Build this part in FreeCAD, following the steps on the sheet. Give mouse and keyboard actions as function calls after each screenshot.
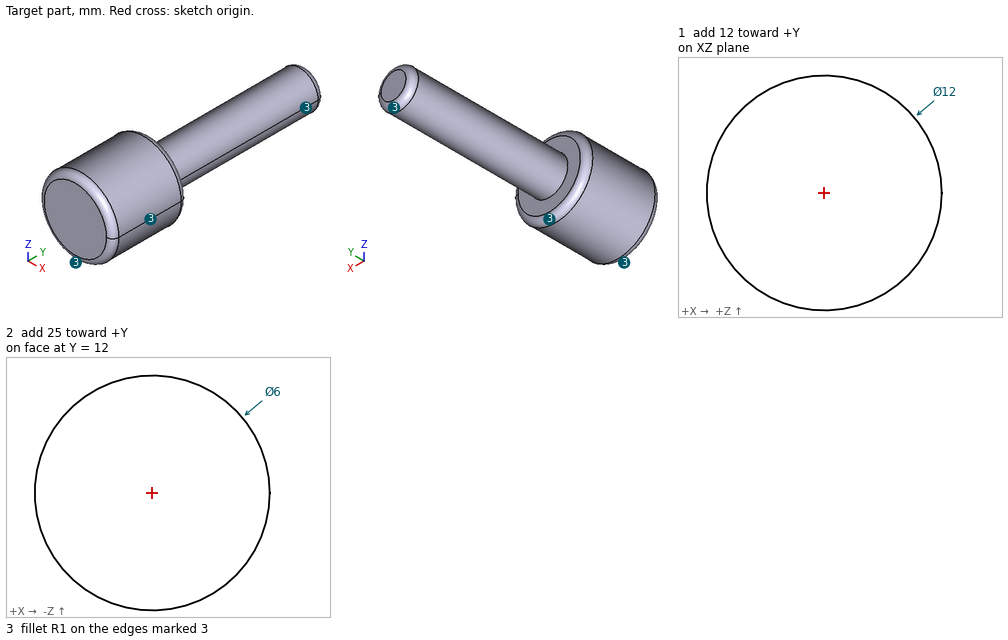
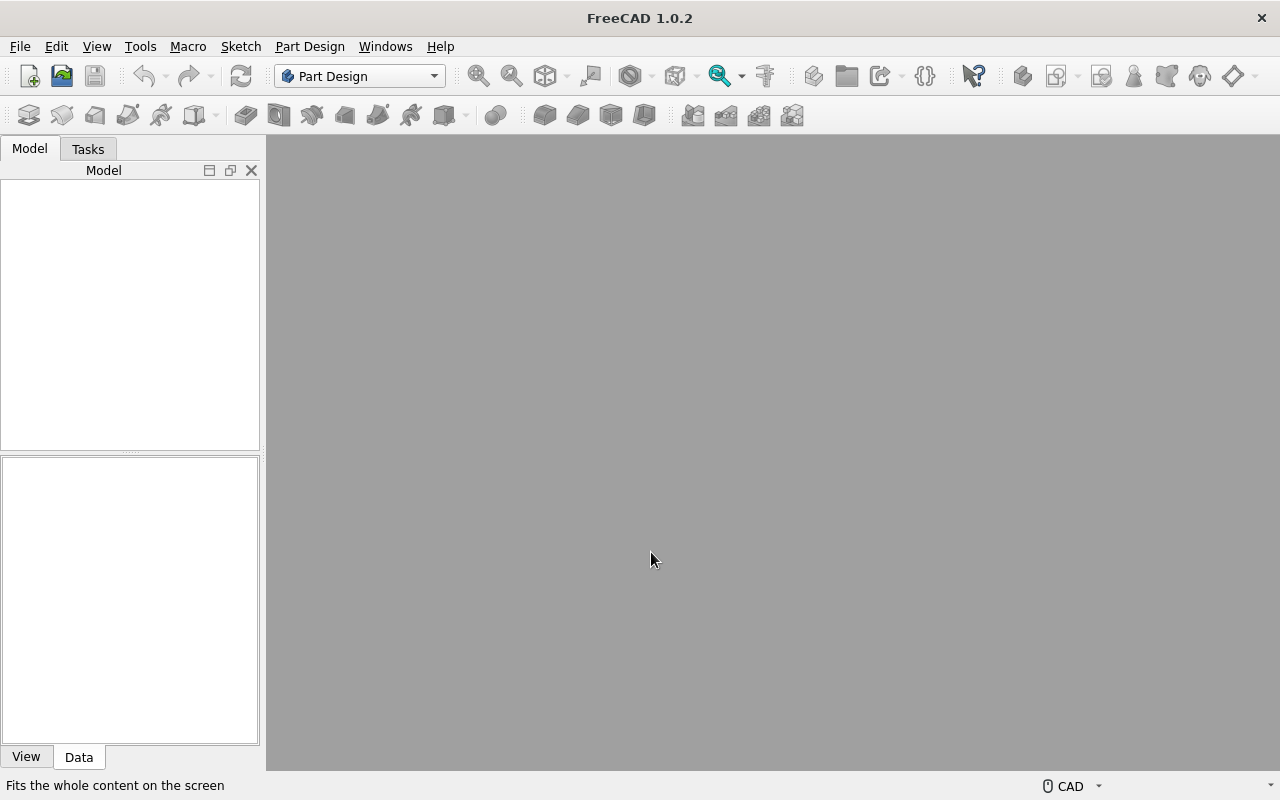
click(29, 76)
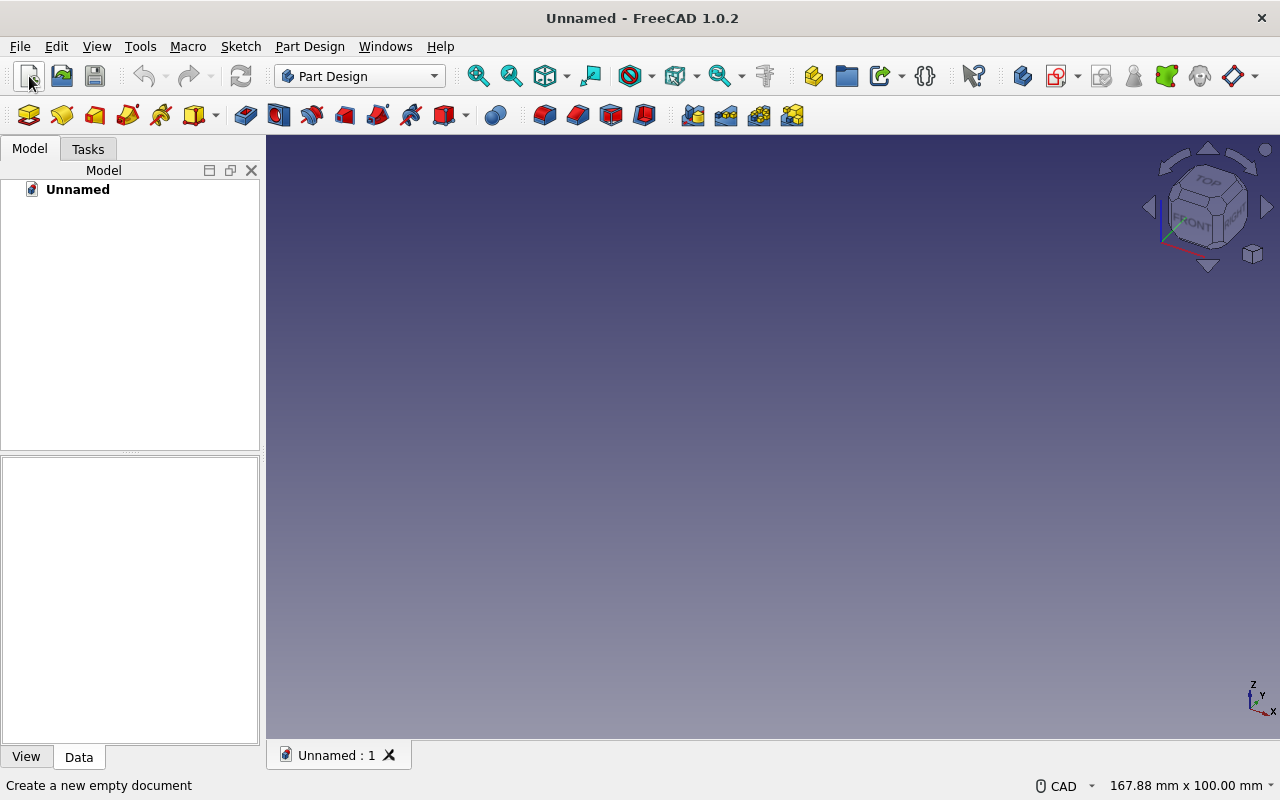
click(1056, 76)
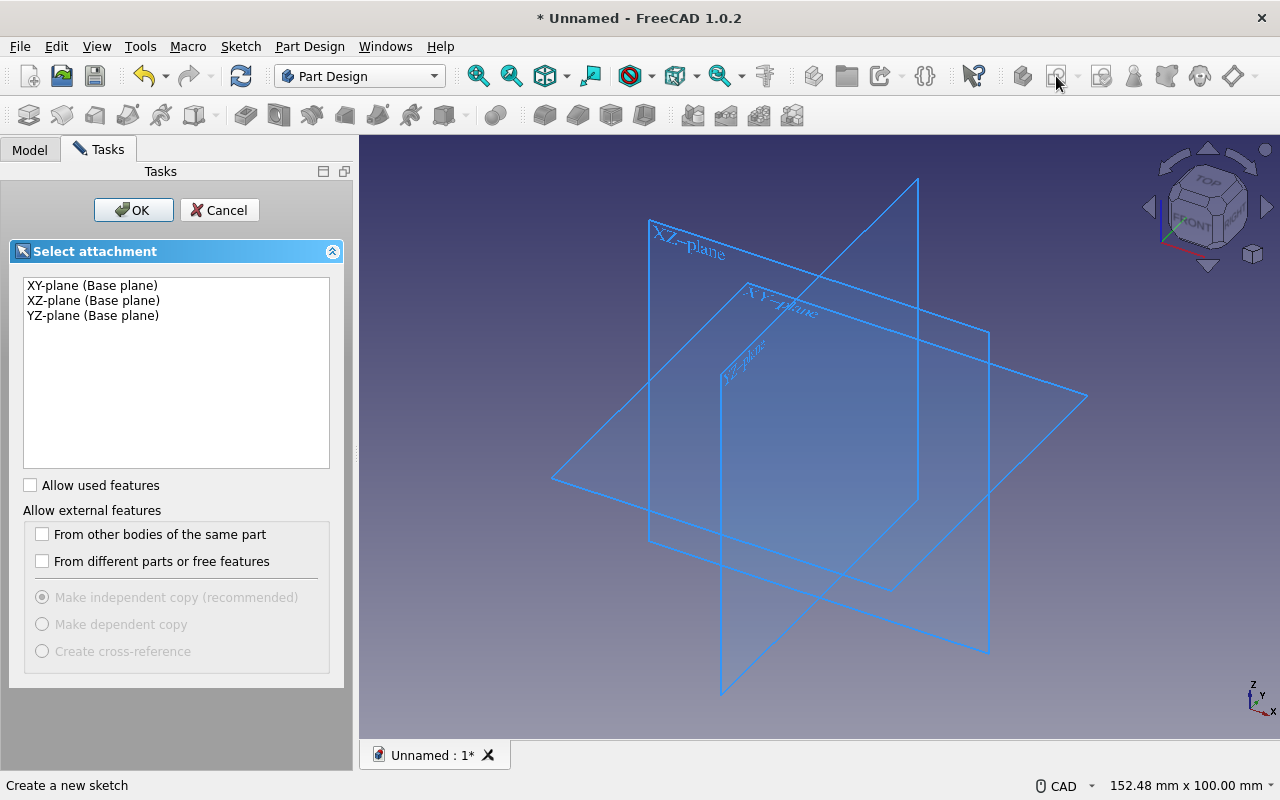
click(84, 300)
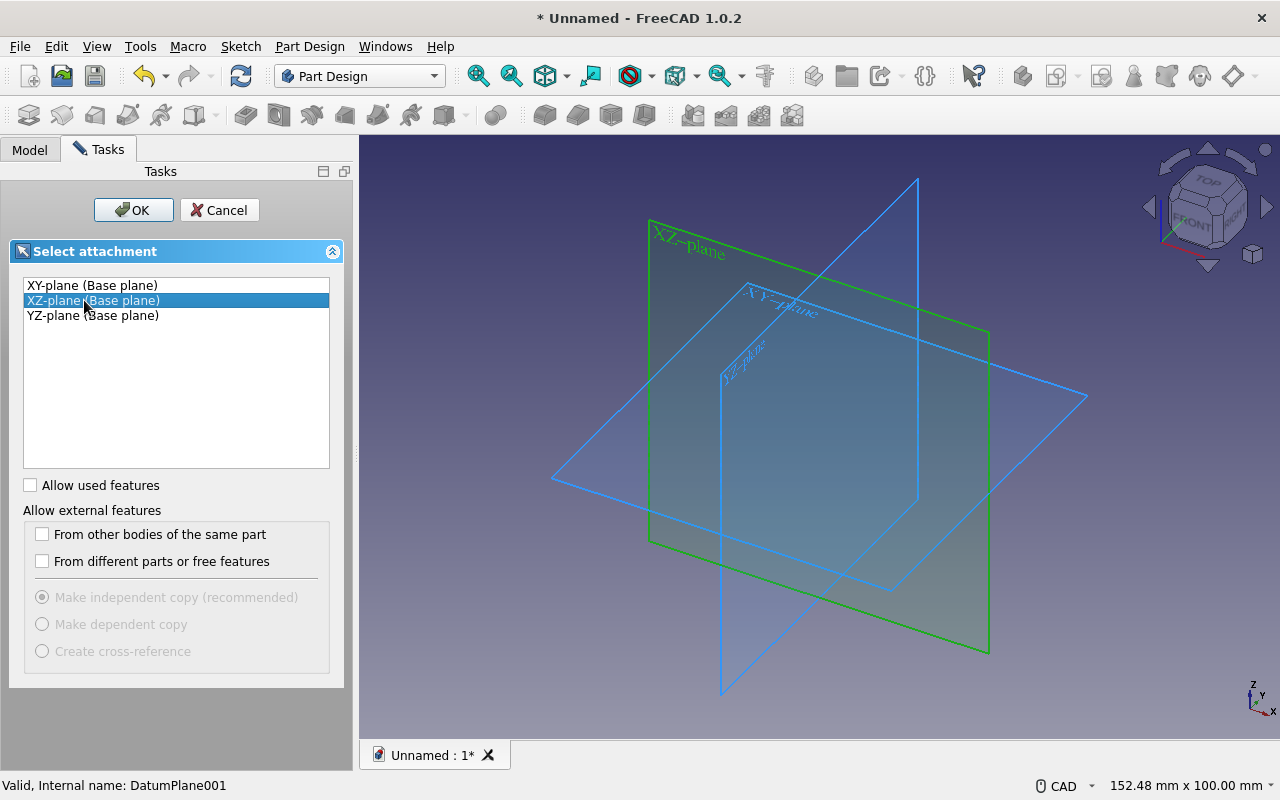
click(134, 210)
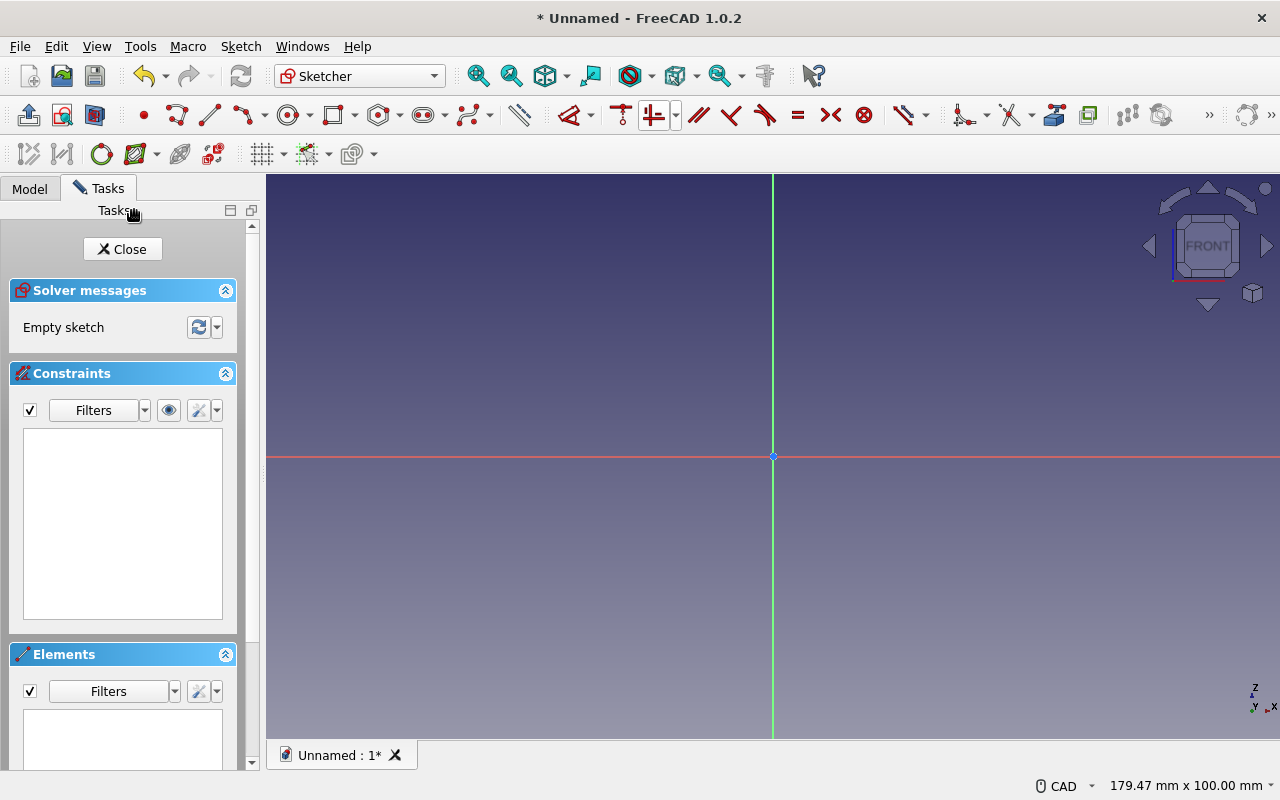
scroll(790, 456, up, 8)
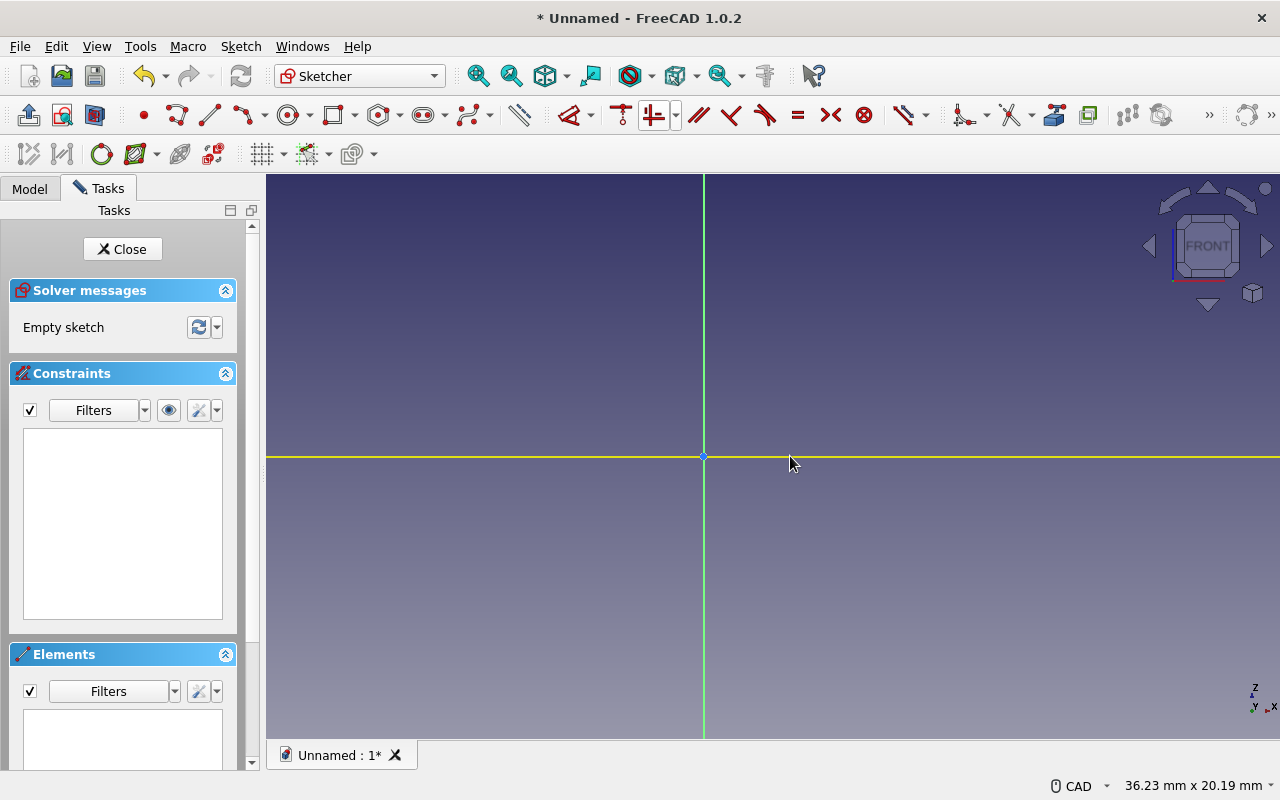
click(288, 116)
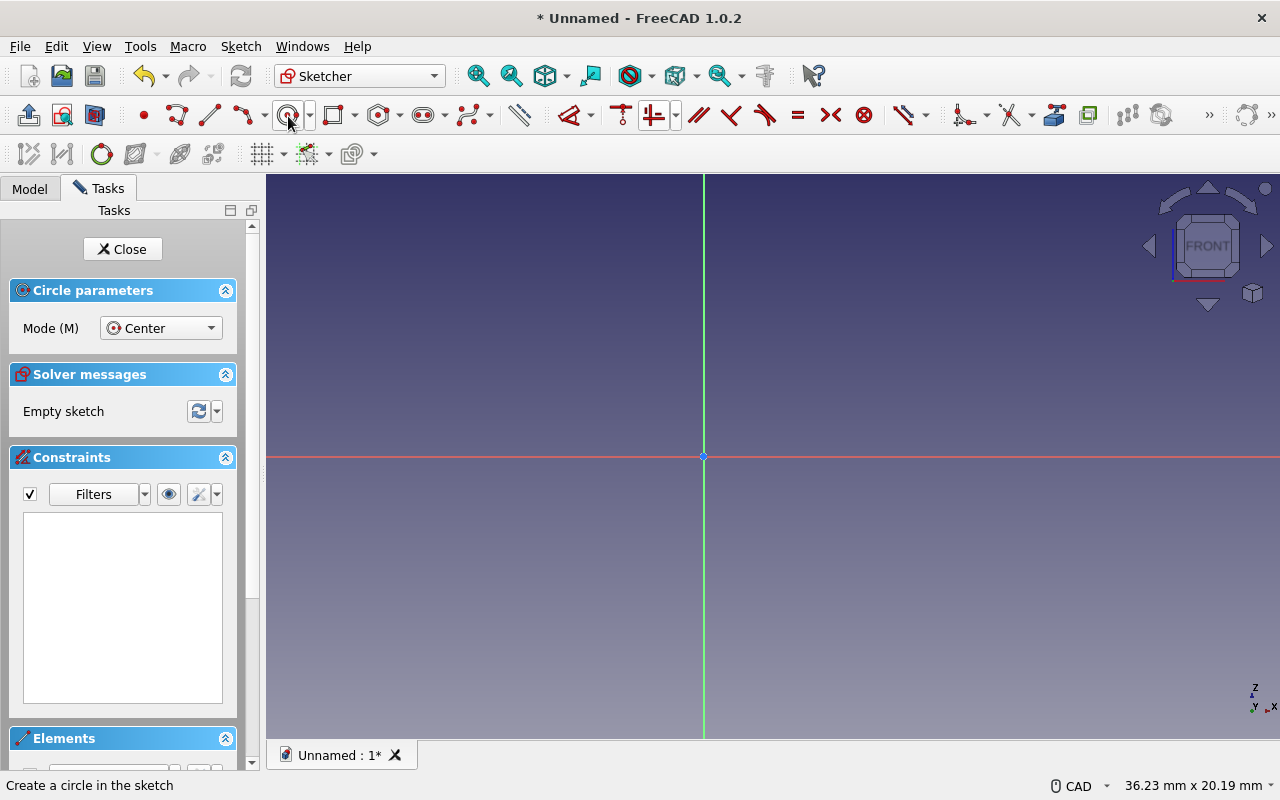
click(704, 456)
move(822, 338)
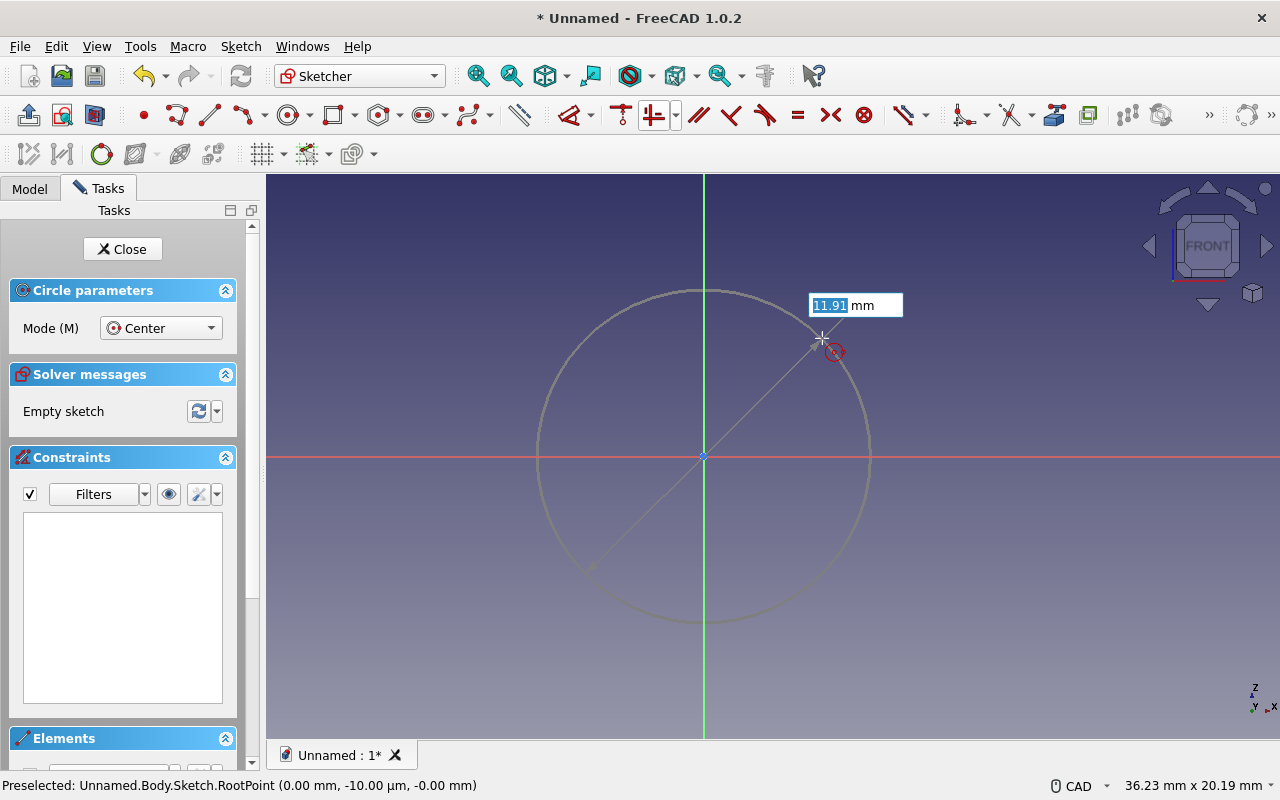
text(12)
key(Return)
key(Escape)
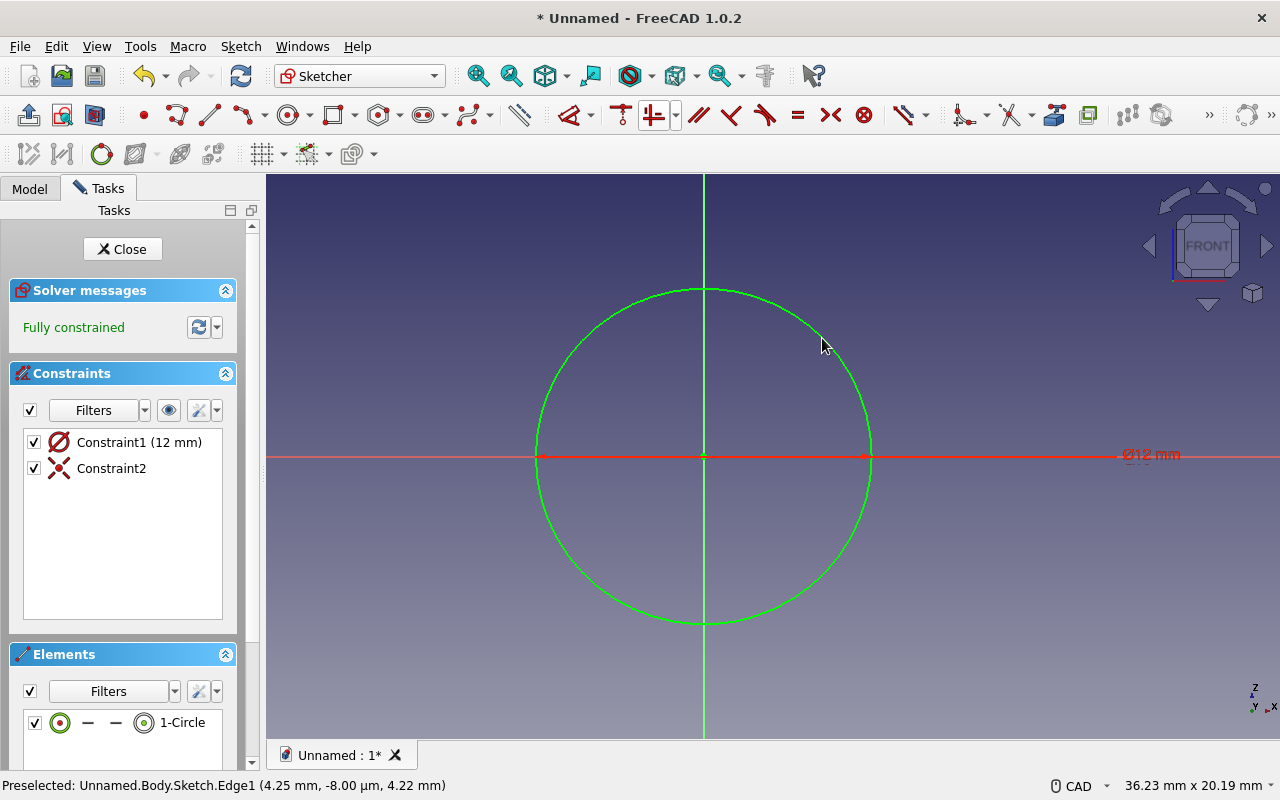
click(123, 249)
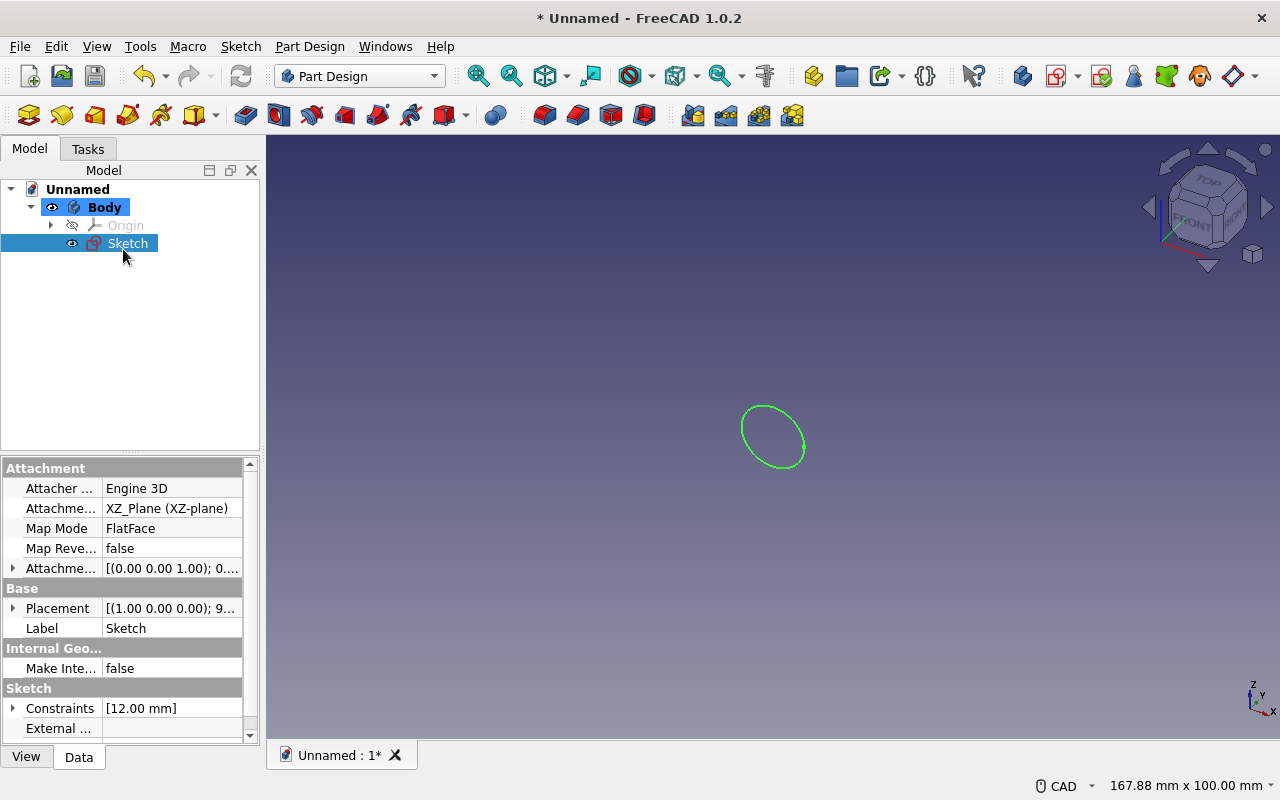
click(29, 116)